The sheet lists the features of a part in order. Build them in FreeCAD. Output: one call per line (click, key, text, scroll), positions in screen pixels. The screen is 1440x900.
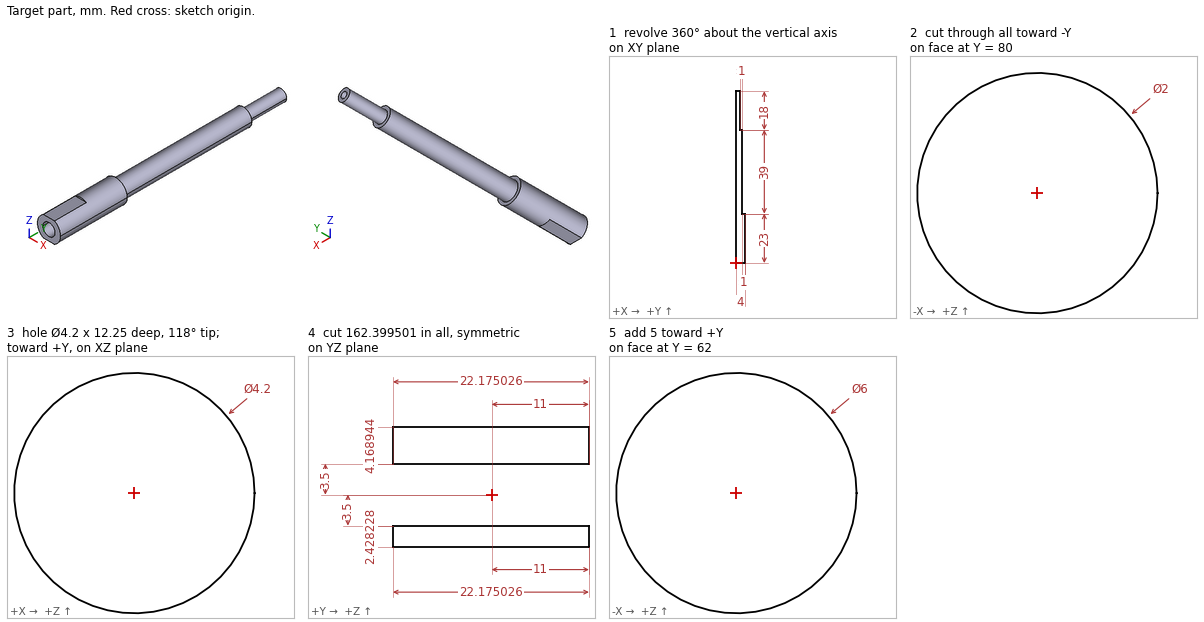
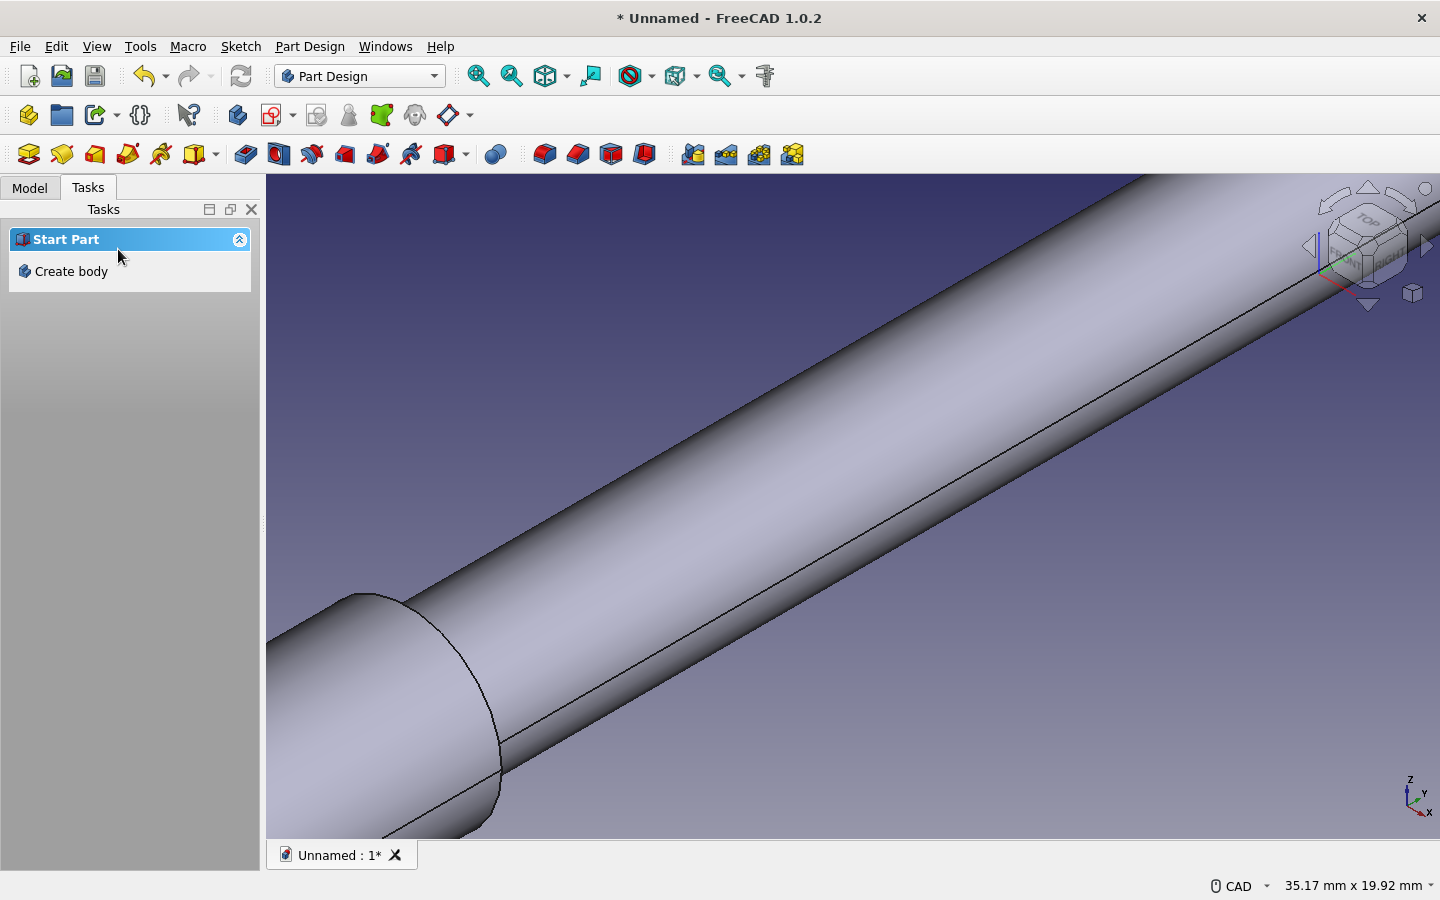
key(v)
key(f)